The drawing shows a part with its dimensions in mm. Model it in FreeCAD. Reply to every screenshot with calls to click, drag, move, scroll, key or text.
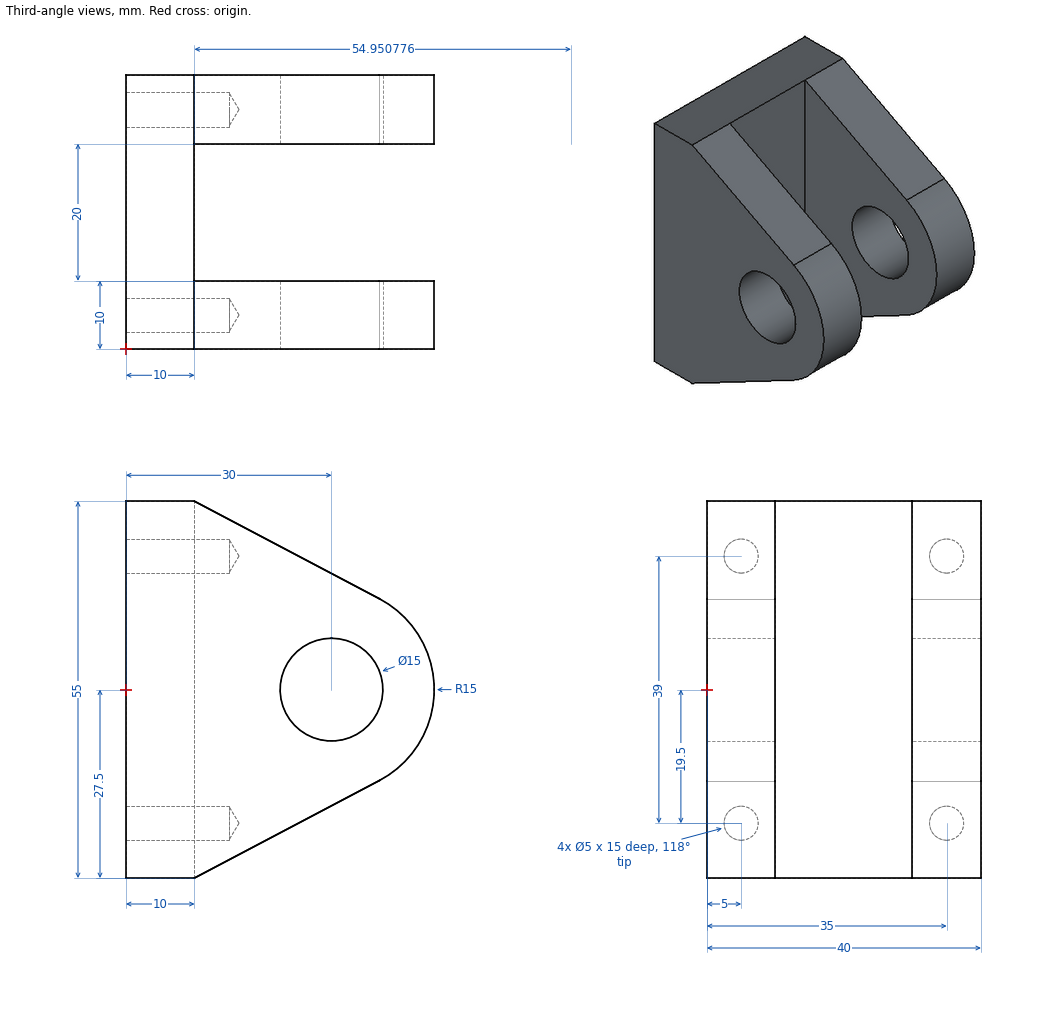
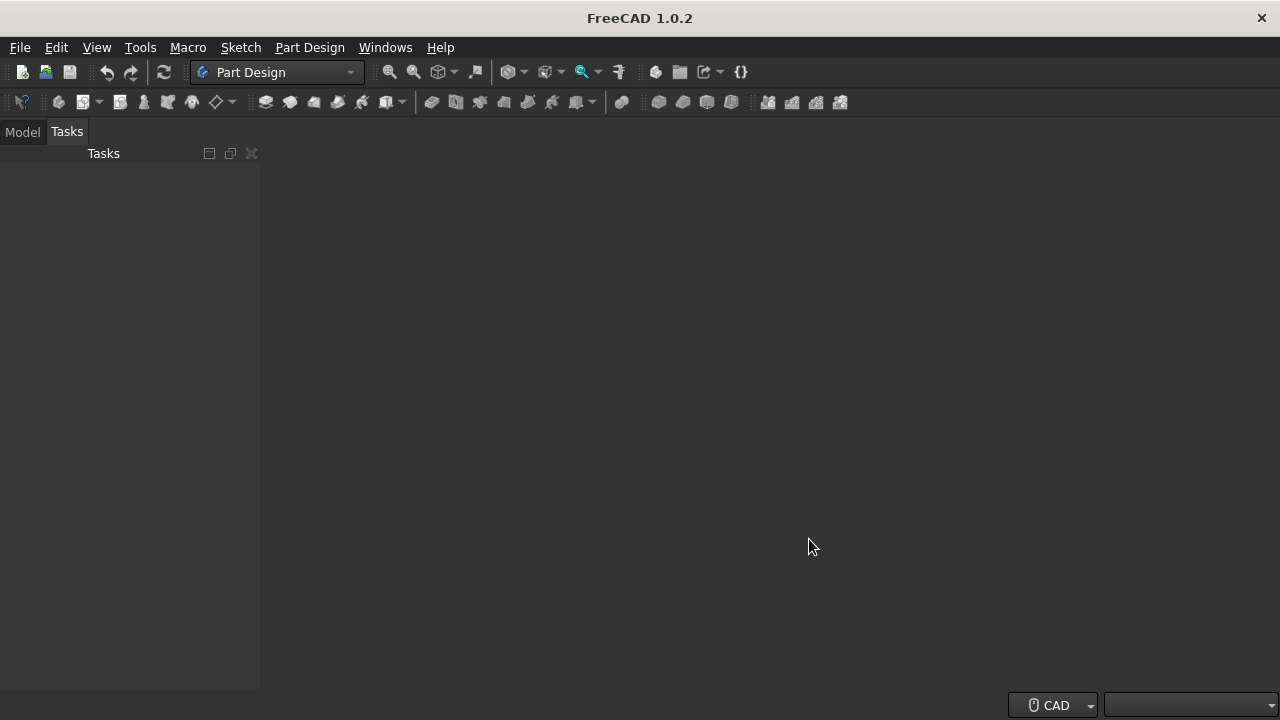
key(ctrl+n)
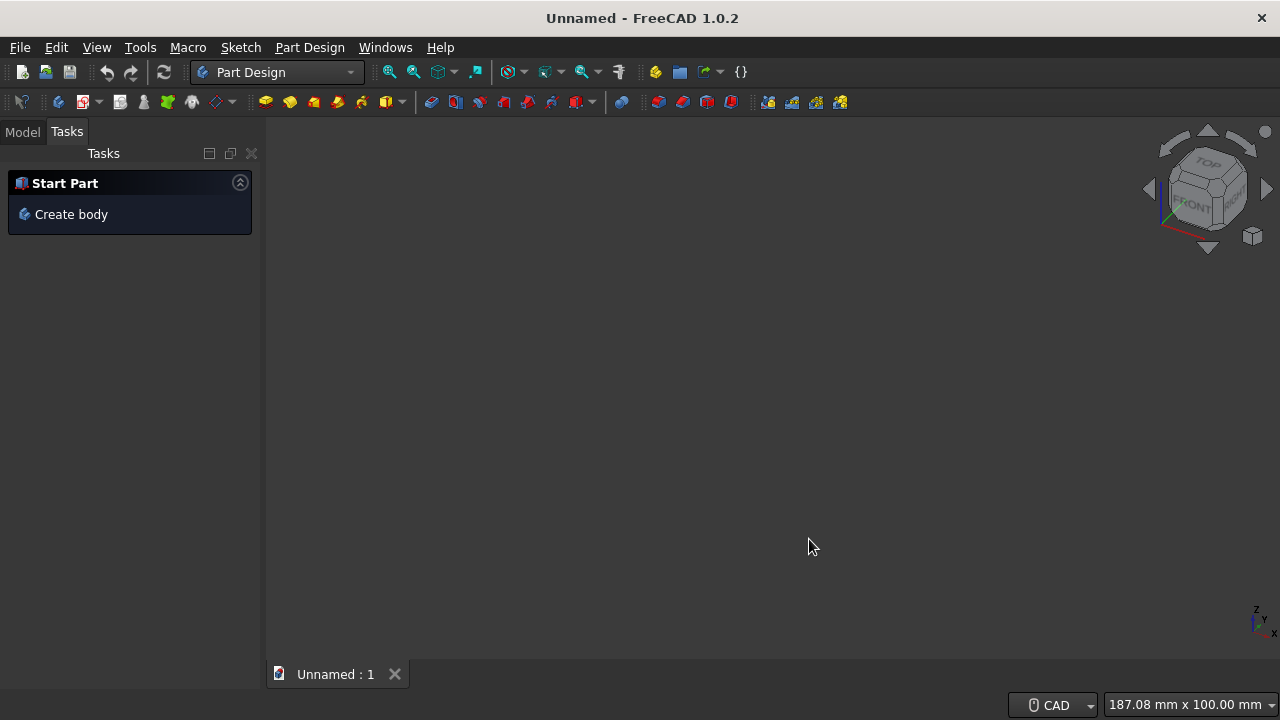
click(84, 102)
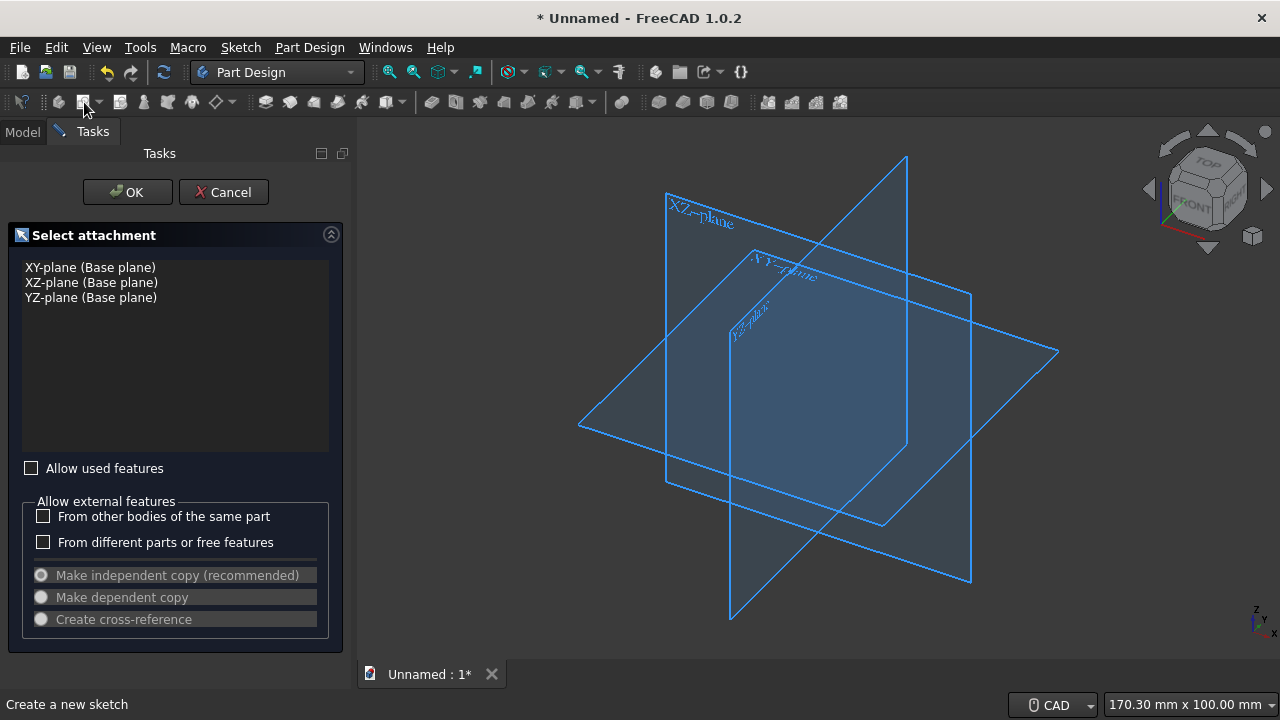
click(82, 282)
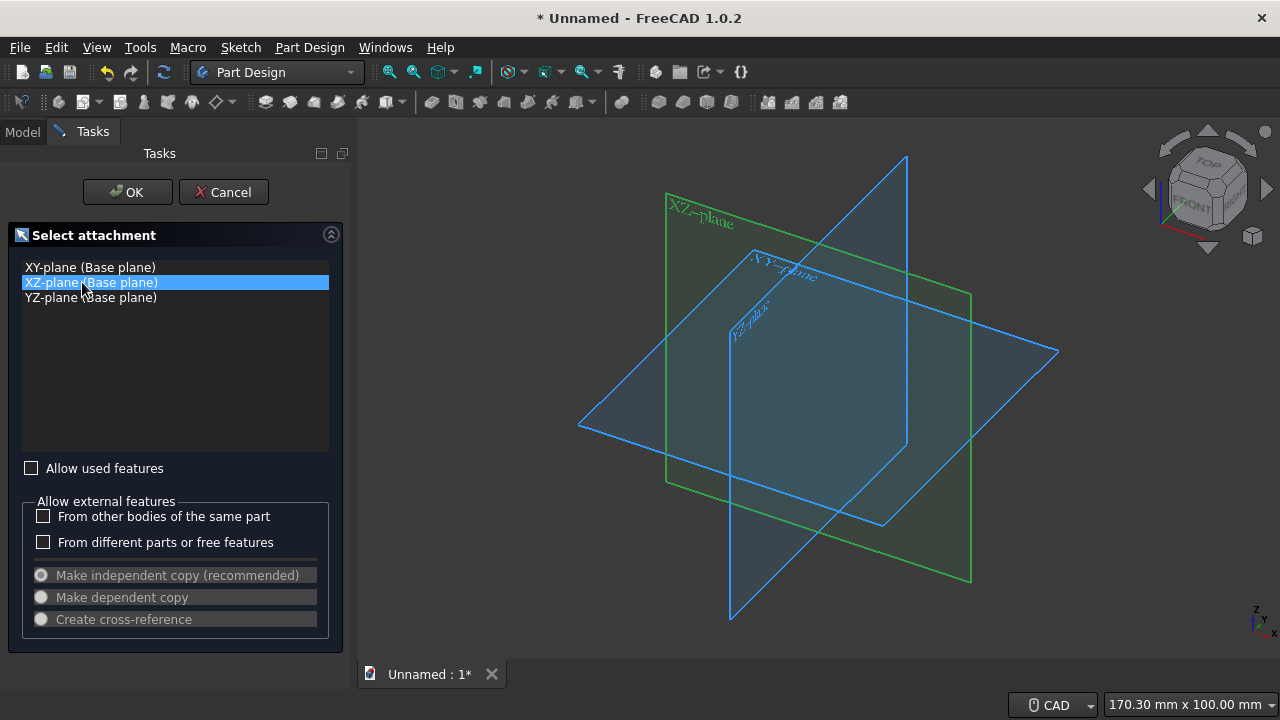
click(128, 192)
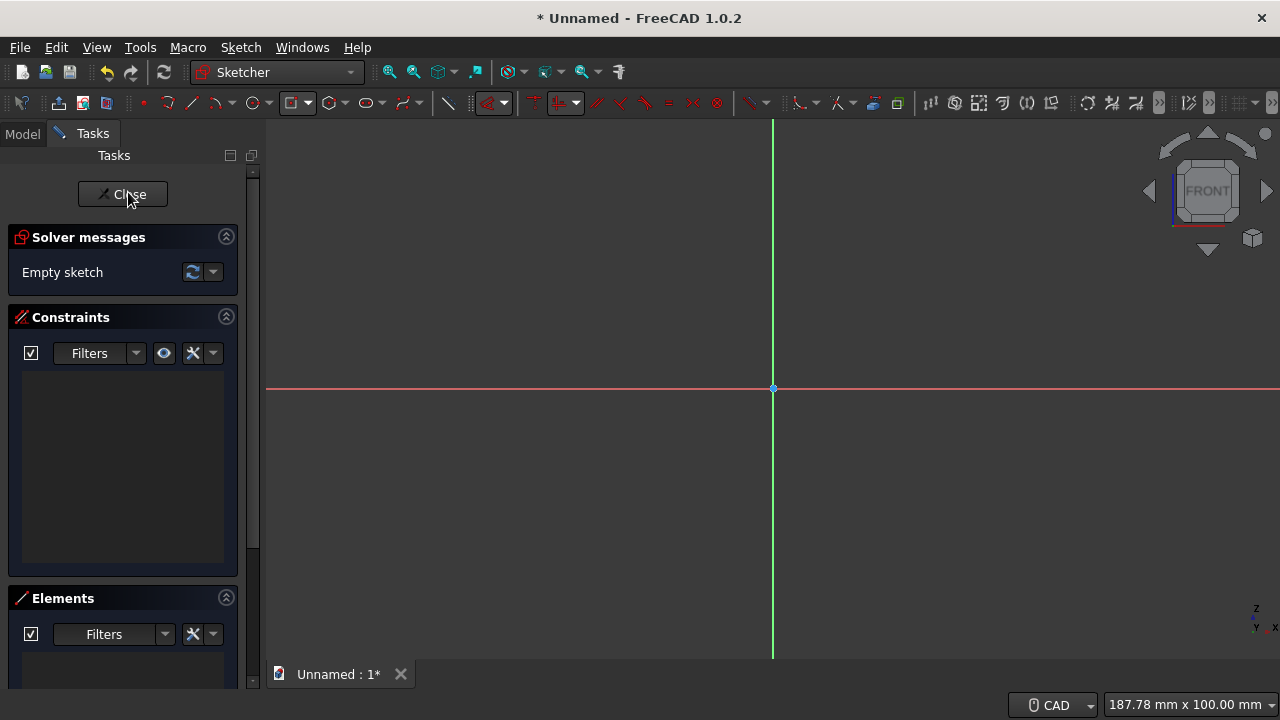
key(g)
key(m)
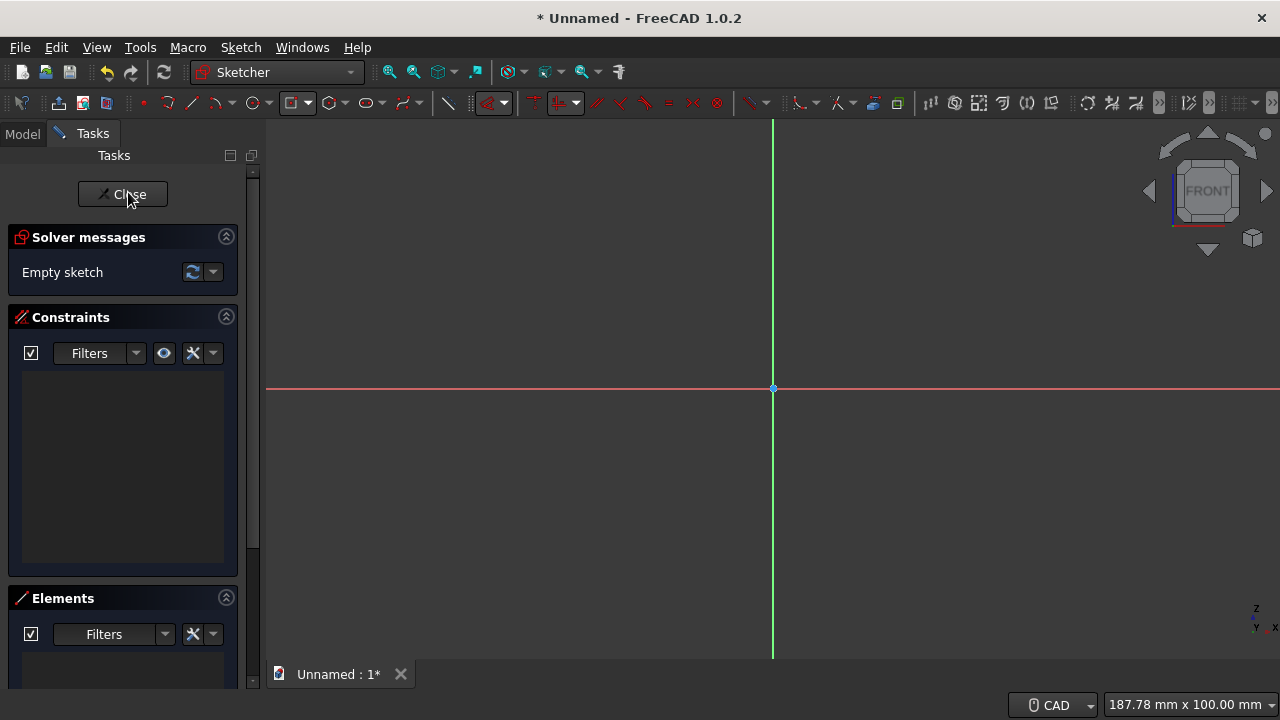
click(973, 461)
click(827, 538)
click(773, 538)
click(782, 241)
click(827, 241)
click(973, 317)
right_click(973, 317)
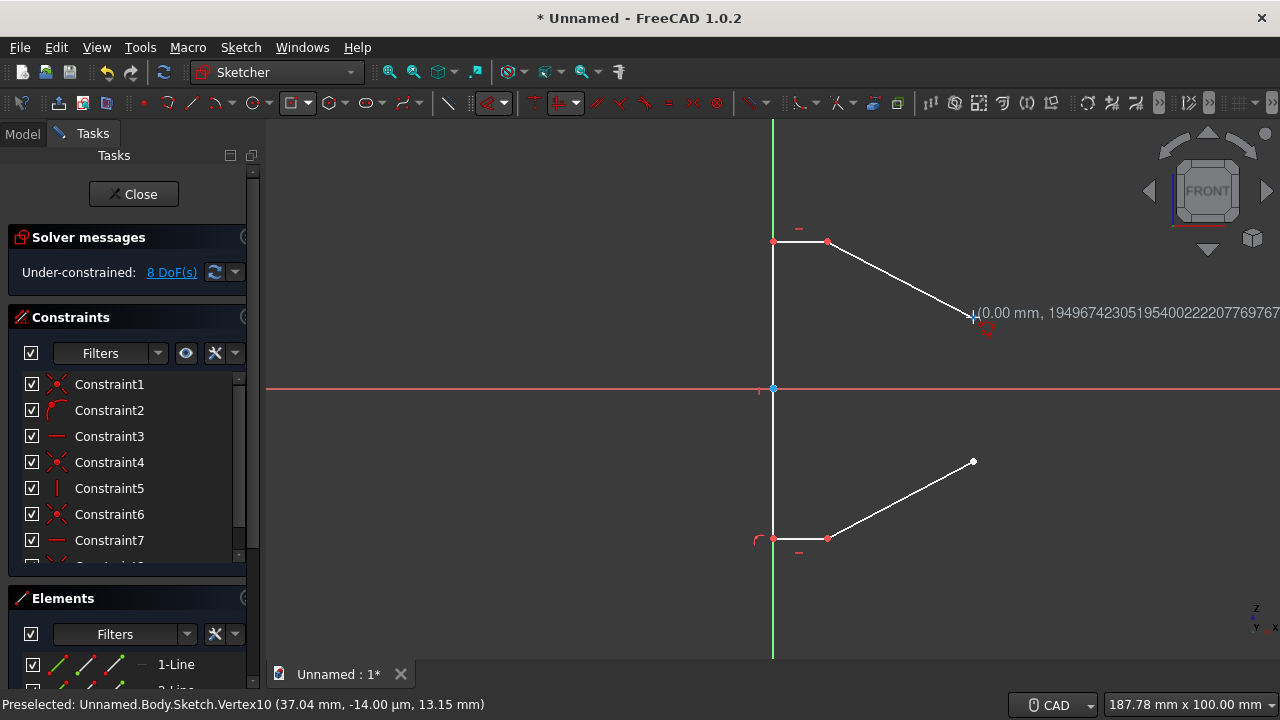
click(234, 104)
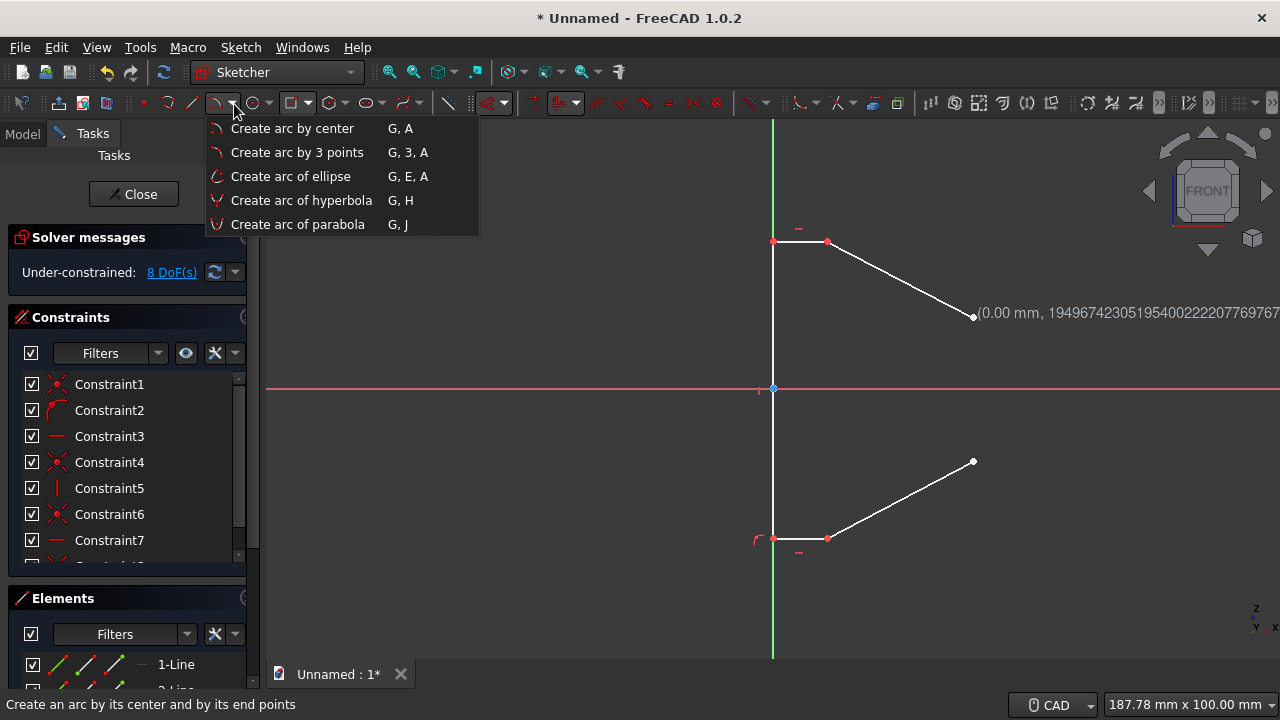
click(342, 152)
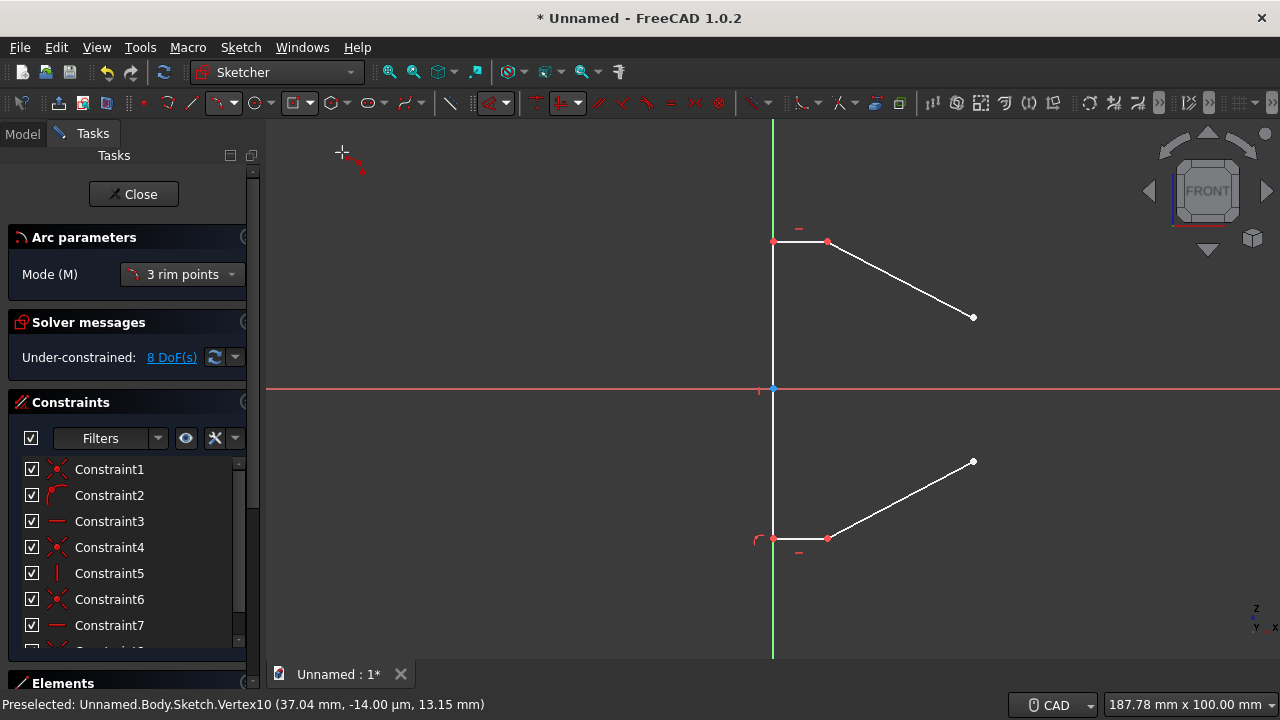
click(973, 318)
click(973, 462)
click(1014, 406)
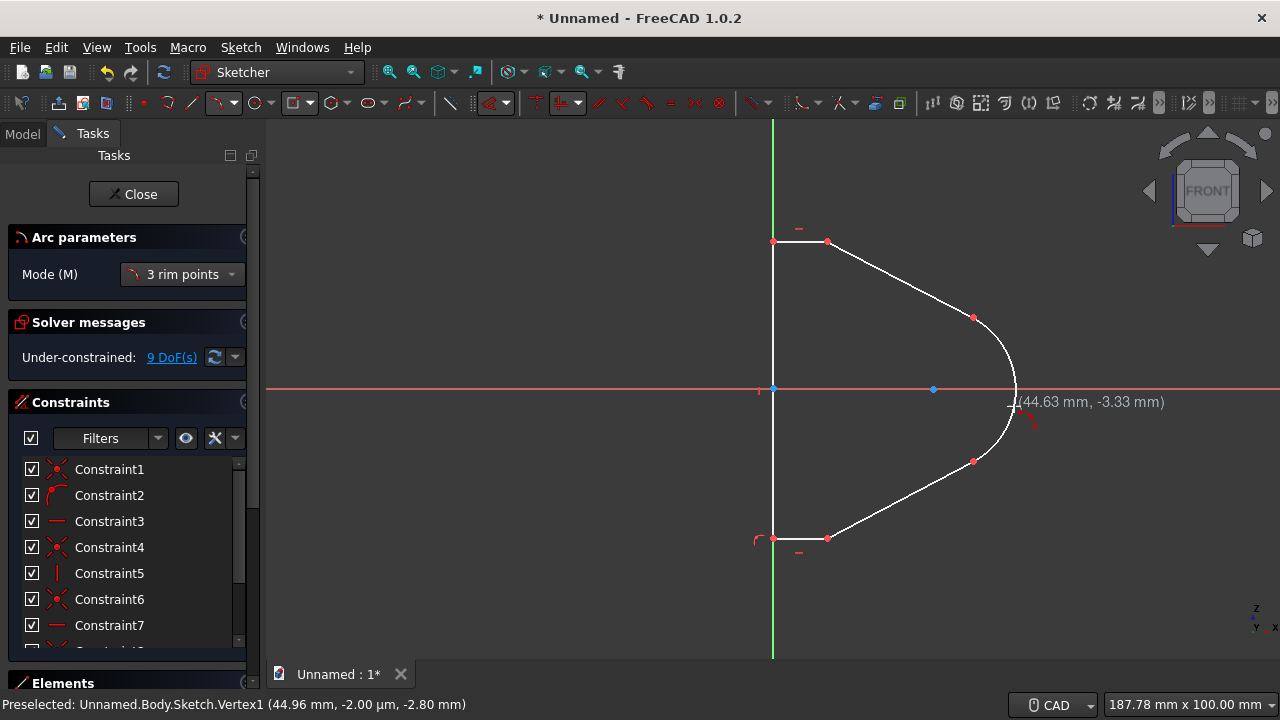
click(256, 104)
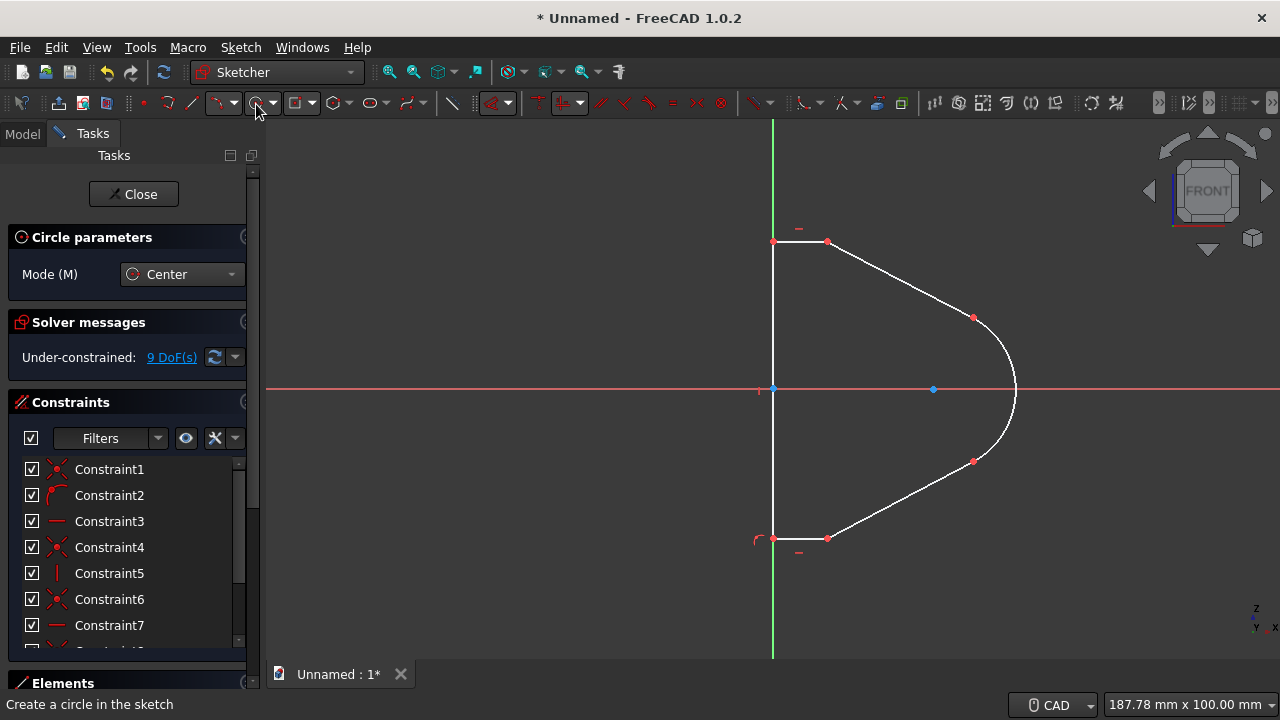
click(935, 389)
click(964, 360)
key(Escape)